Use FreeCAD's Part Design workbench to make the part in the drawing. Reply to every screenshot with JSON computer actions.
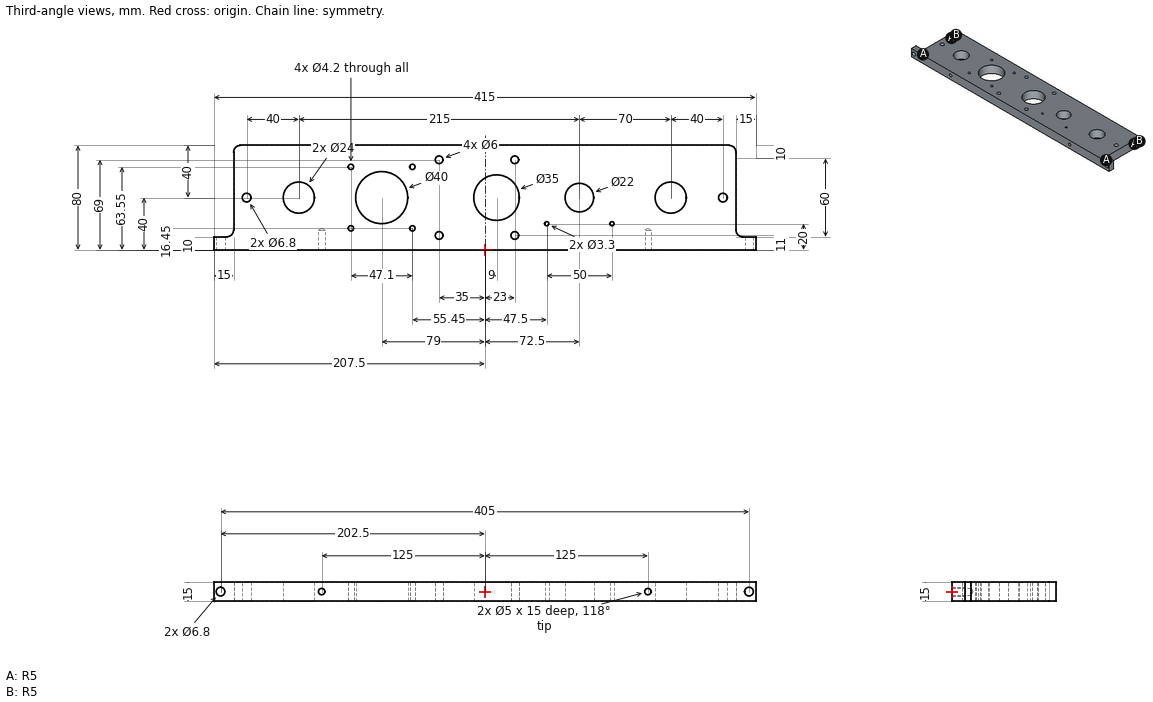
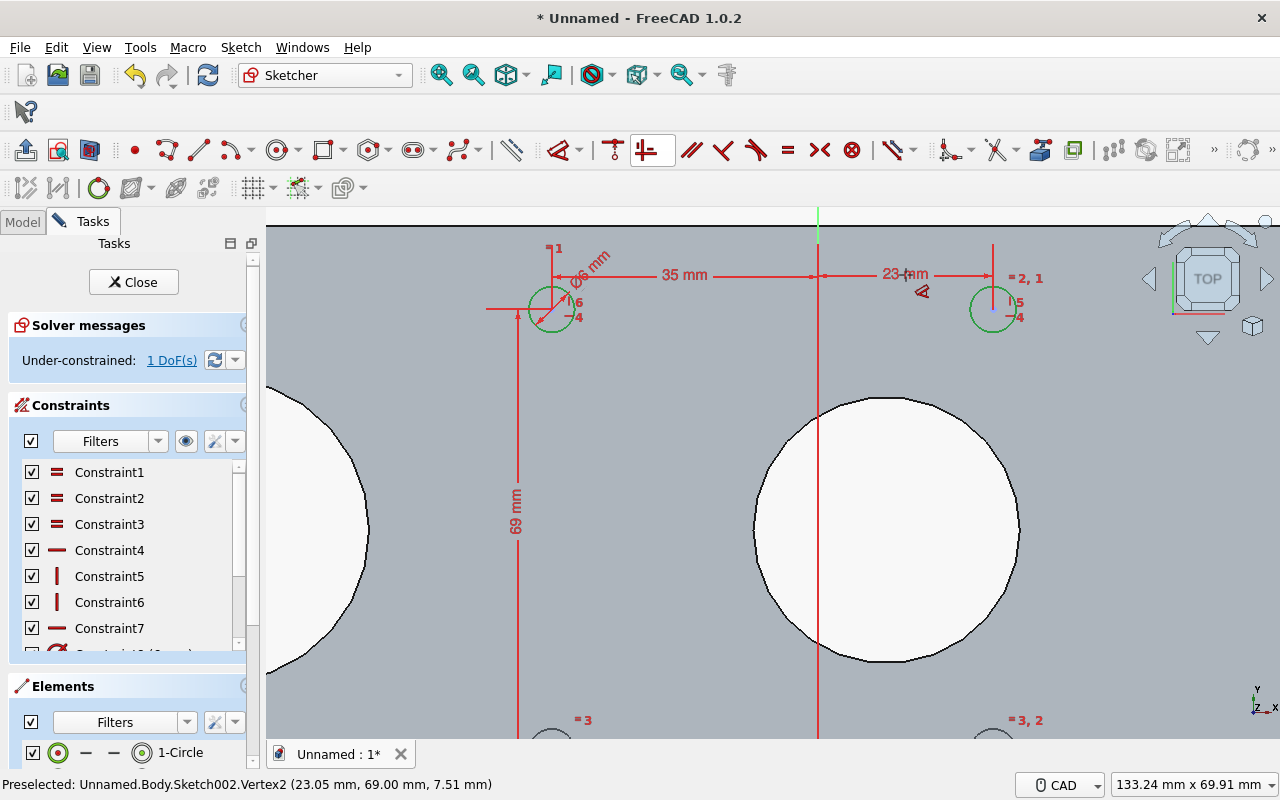
{"action": "scroll", "coordinate": [566, 295], "scroll_direction": "down", "scroll_amount": 2}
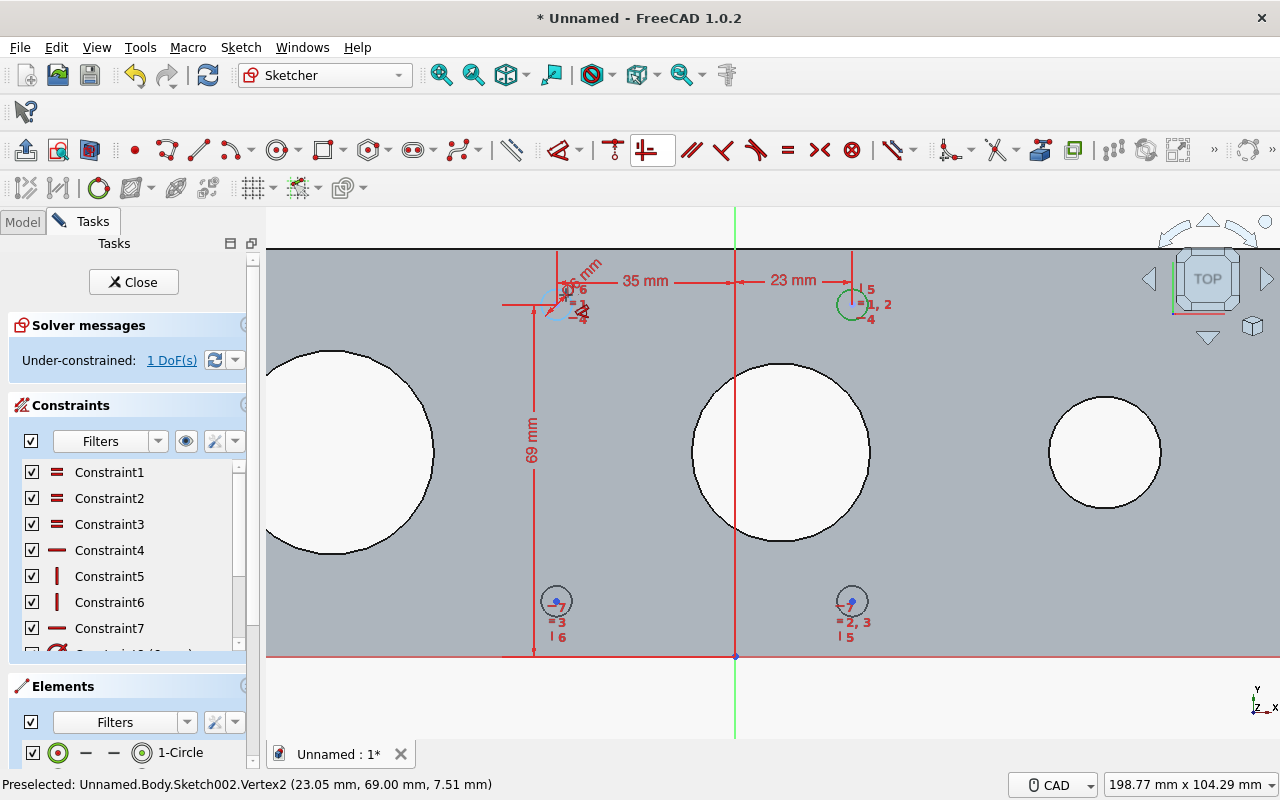
{"action": "left_click", "coordinate": [852, 601]}
{"action": "left_click", "coordinate": [886, 629]}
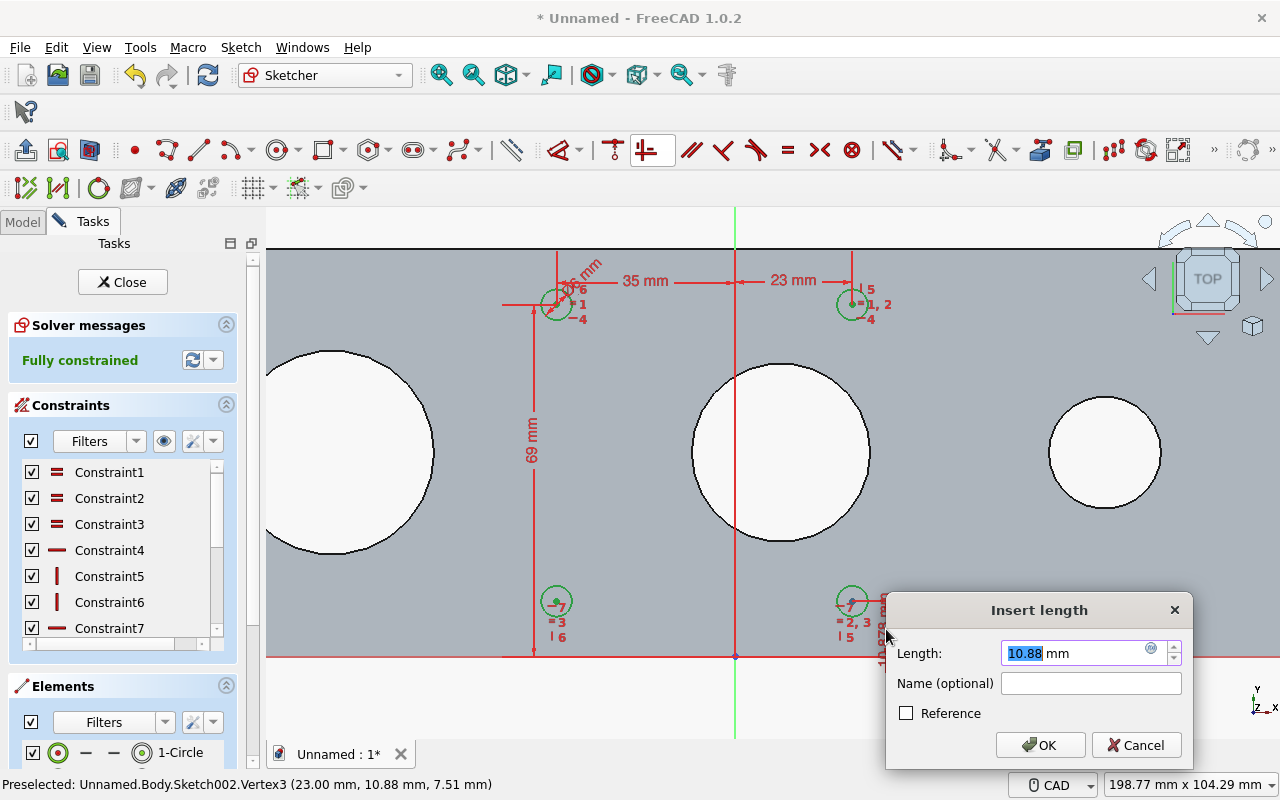
{"action": "type", "text": "11"}
{"action": "key", "text": "Return"}
{"action": "key", "text": "Escape"}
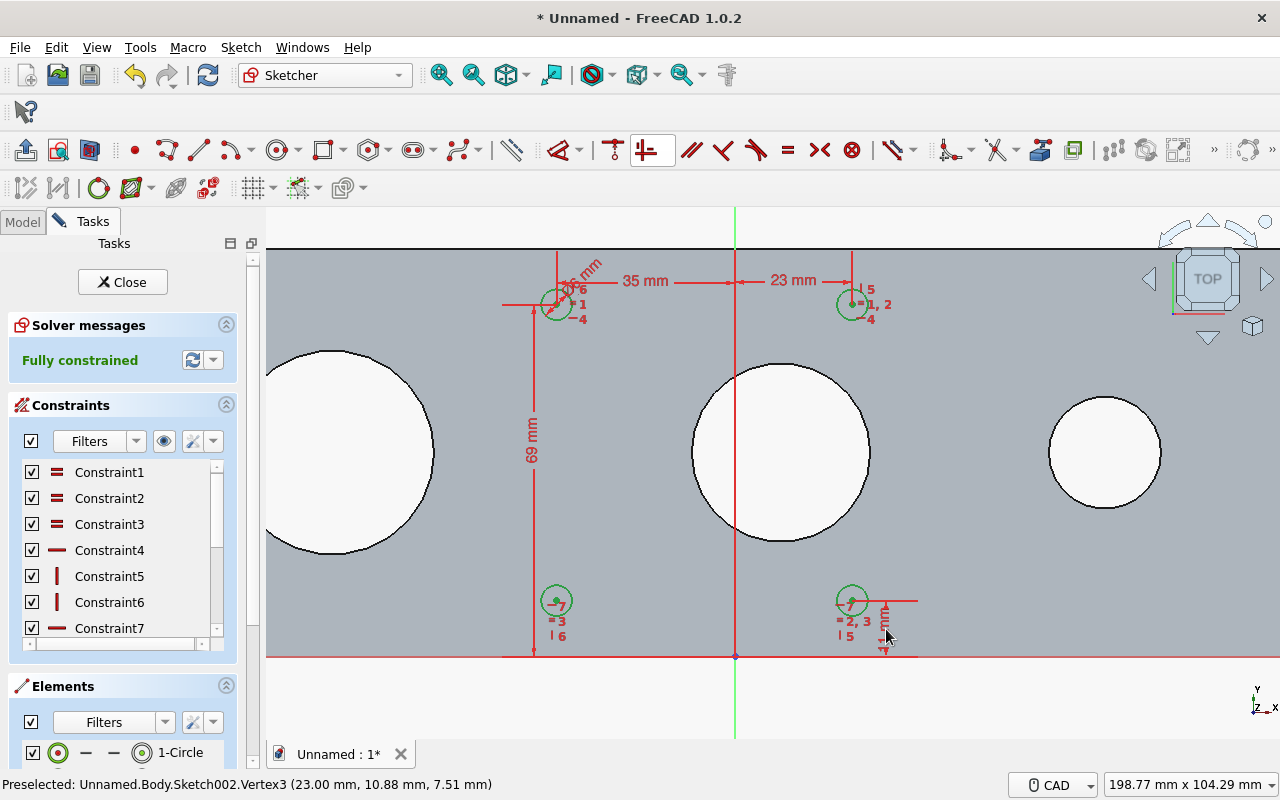
{"action": "left_click", "coordinate": [123, 282]}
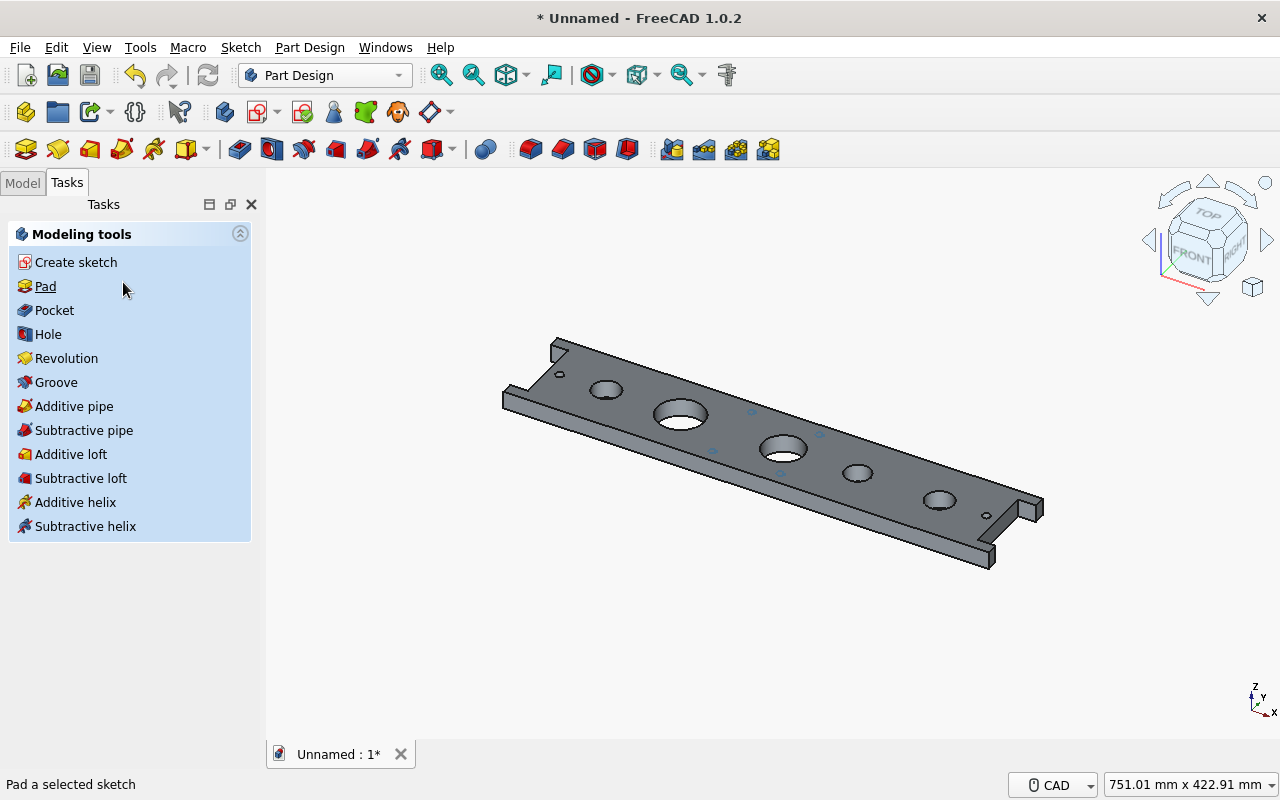
{"action": "left_click", "coordinate": [240, 150]}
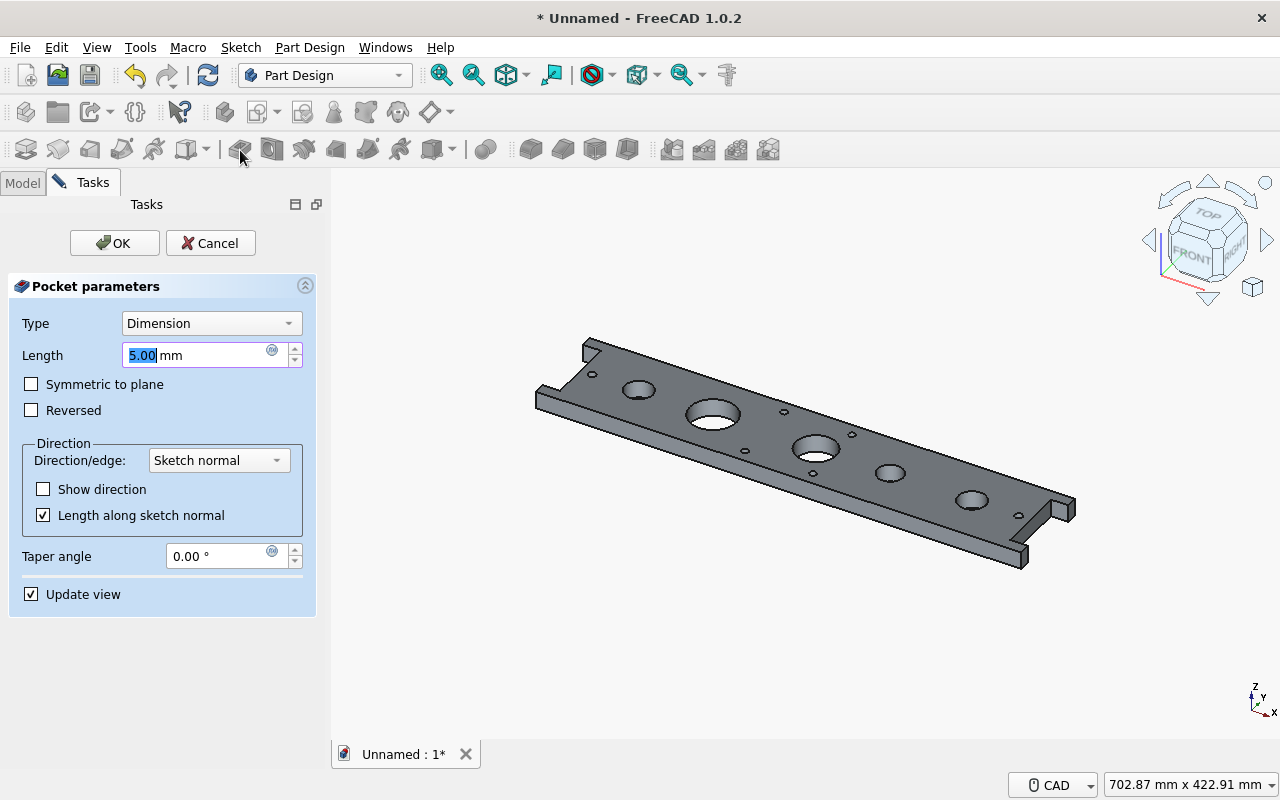
{"action": "type", "text": "15"}
{"action": "key", "text": "Tab"}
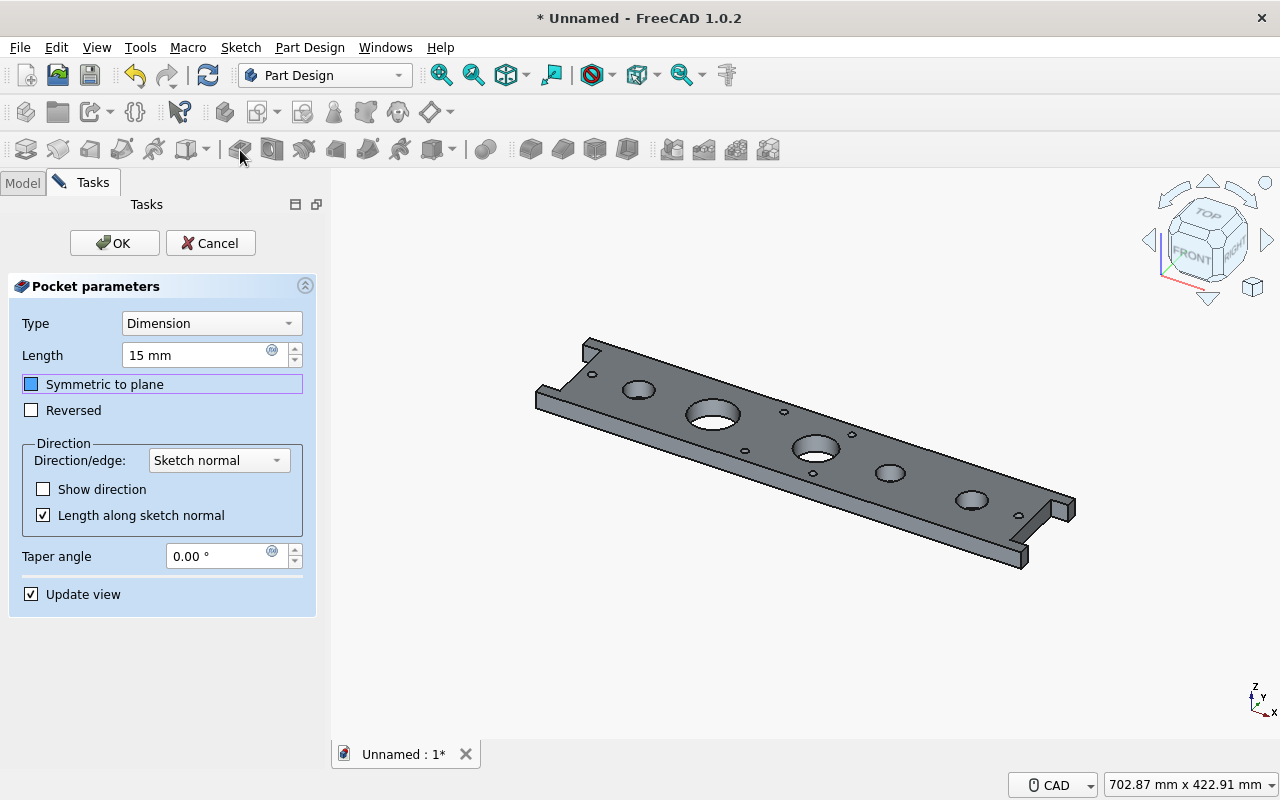
{"action": "left_click", "coordinate": [115, 243]}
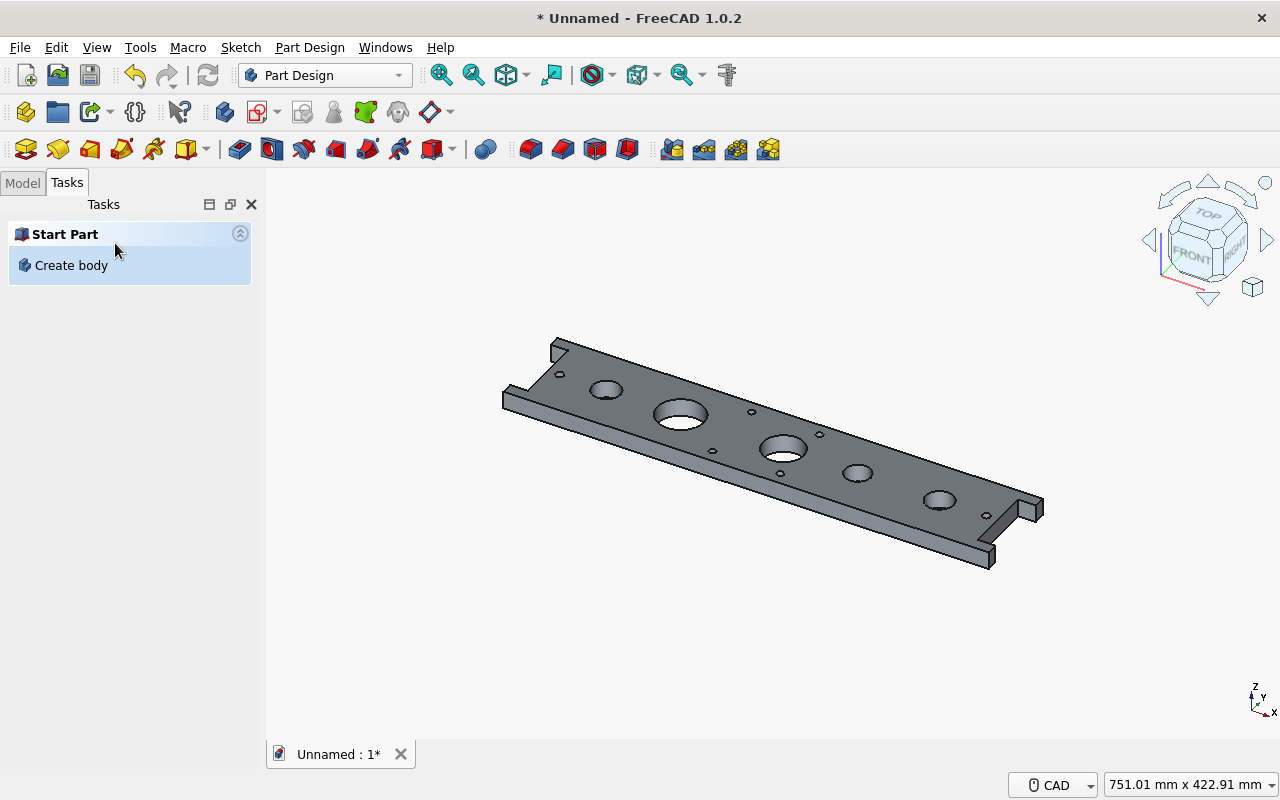
{"action": "key", "text": "4"}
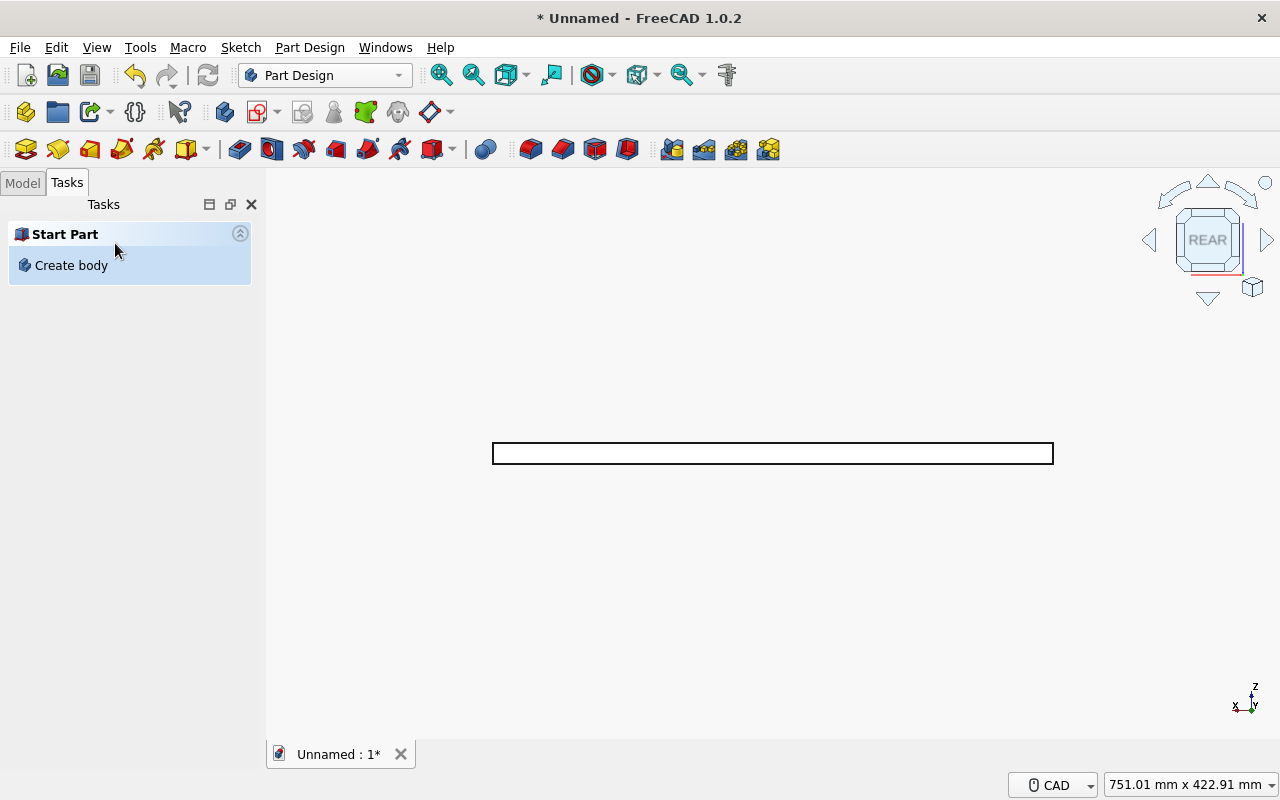
{"action": "left_click", "coordinate": [533, 452]}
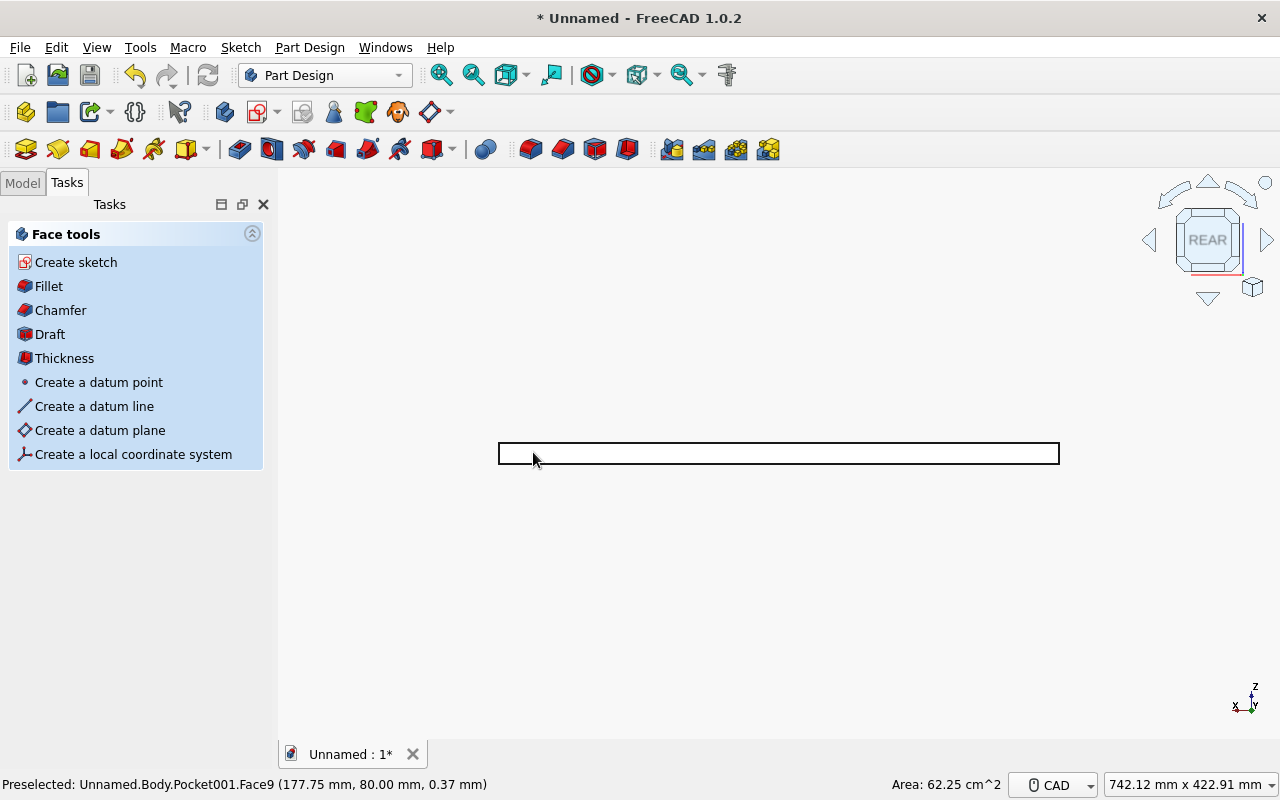
{"action": "left_click", "coordinate": [258, 112]}